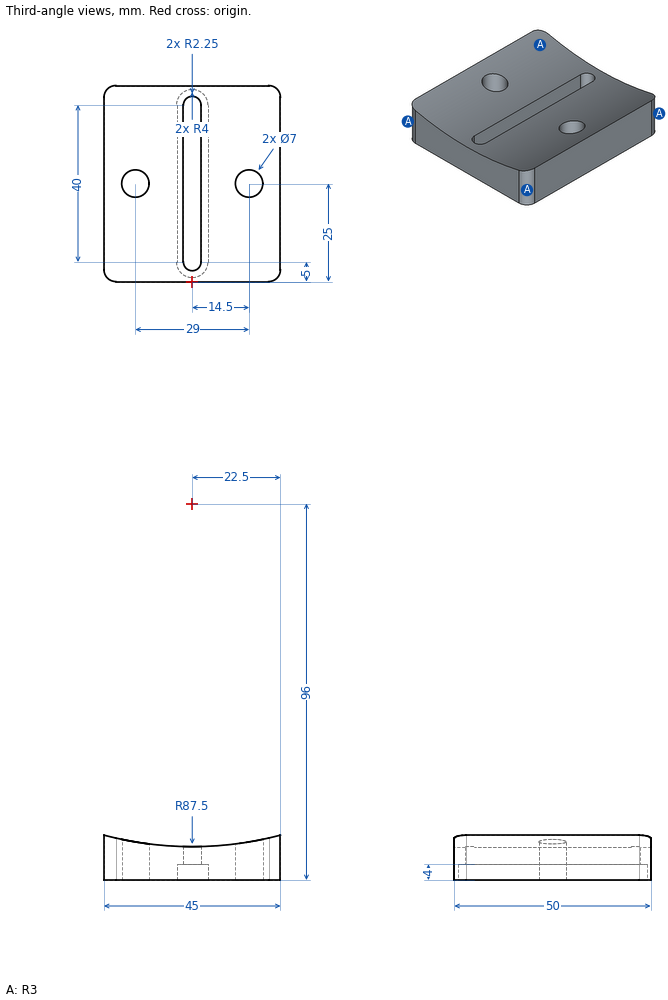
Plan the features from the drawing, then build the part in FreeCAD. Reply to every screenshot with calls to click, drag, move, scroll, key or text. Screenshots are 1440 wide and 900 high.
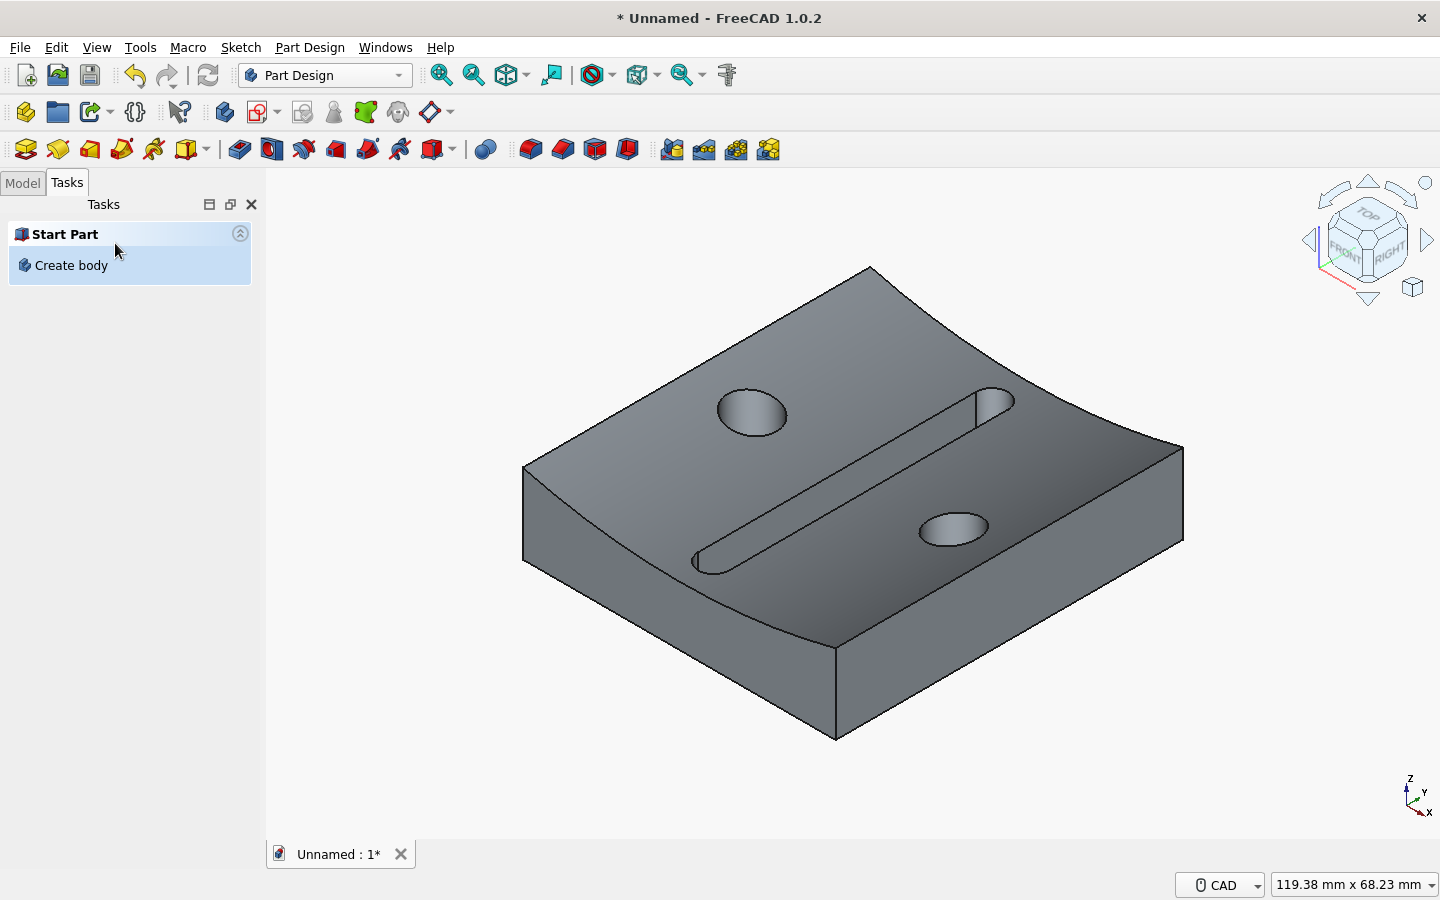
click(836, 693)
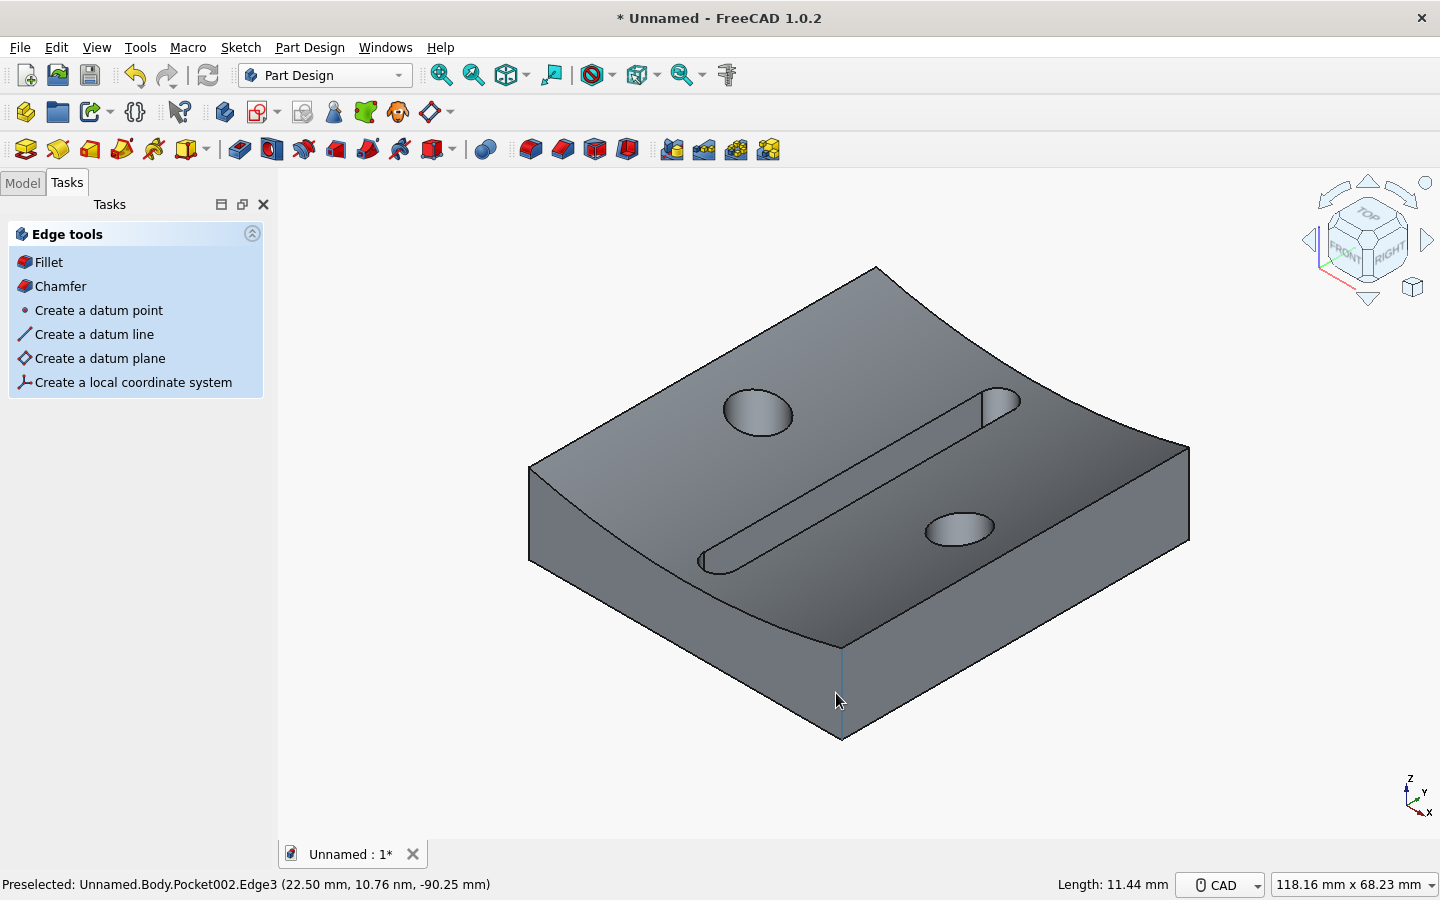
key(2)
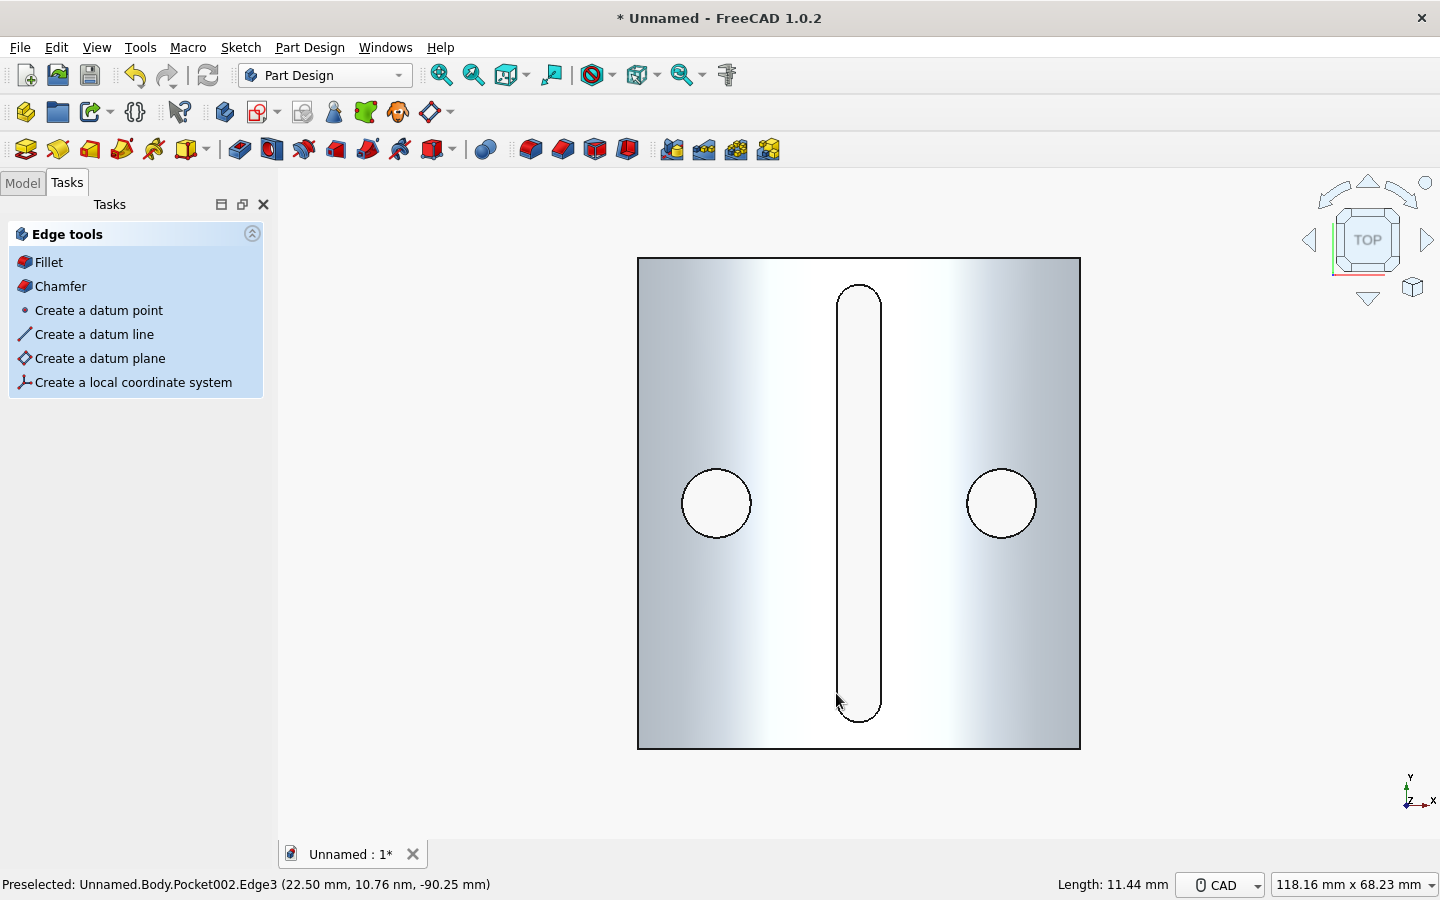
key(1)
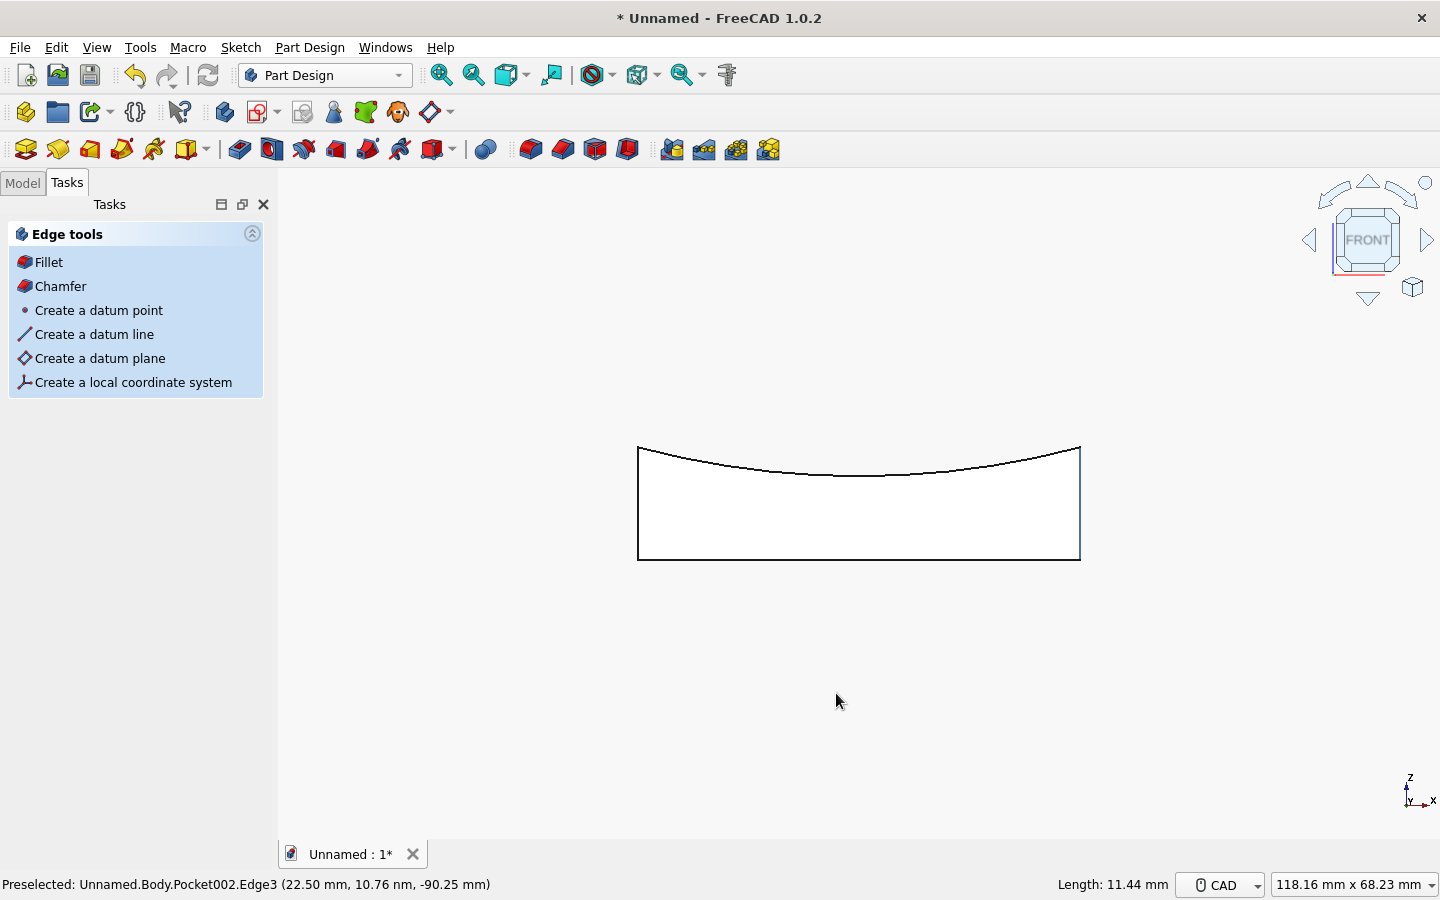
click(442, 76)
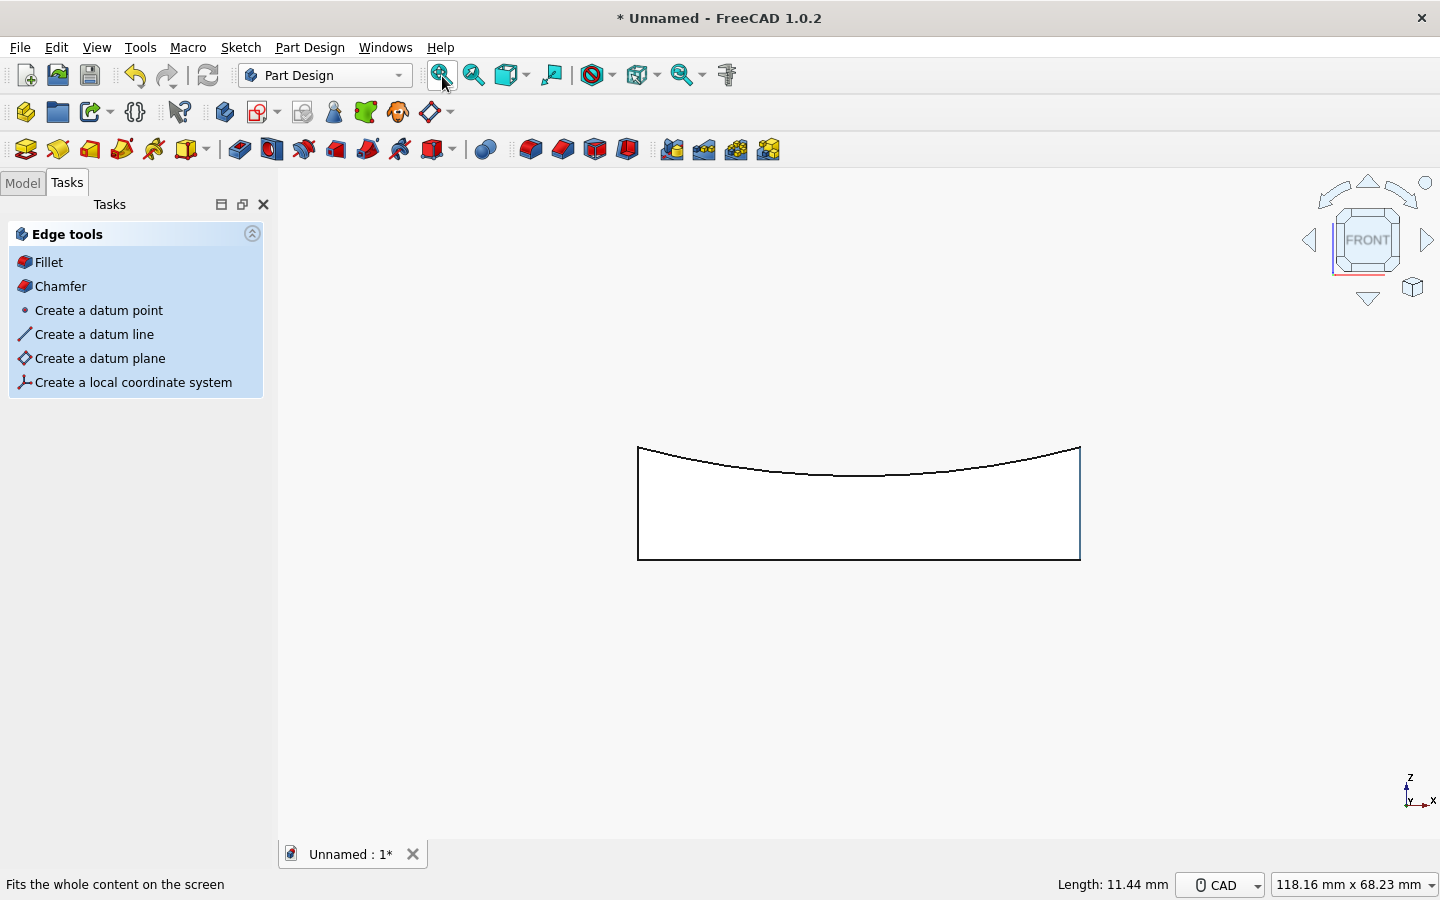
click(638, 502, ctrl)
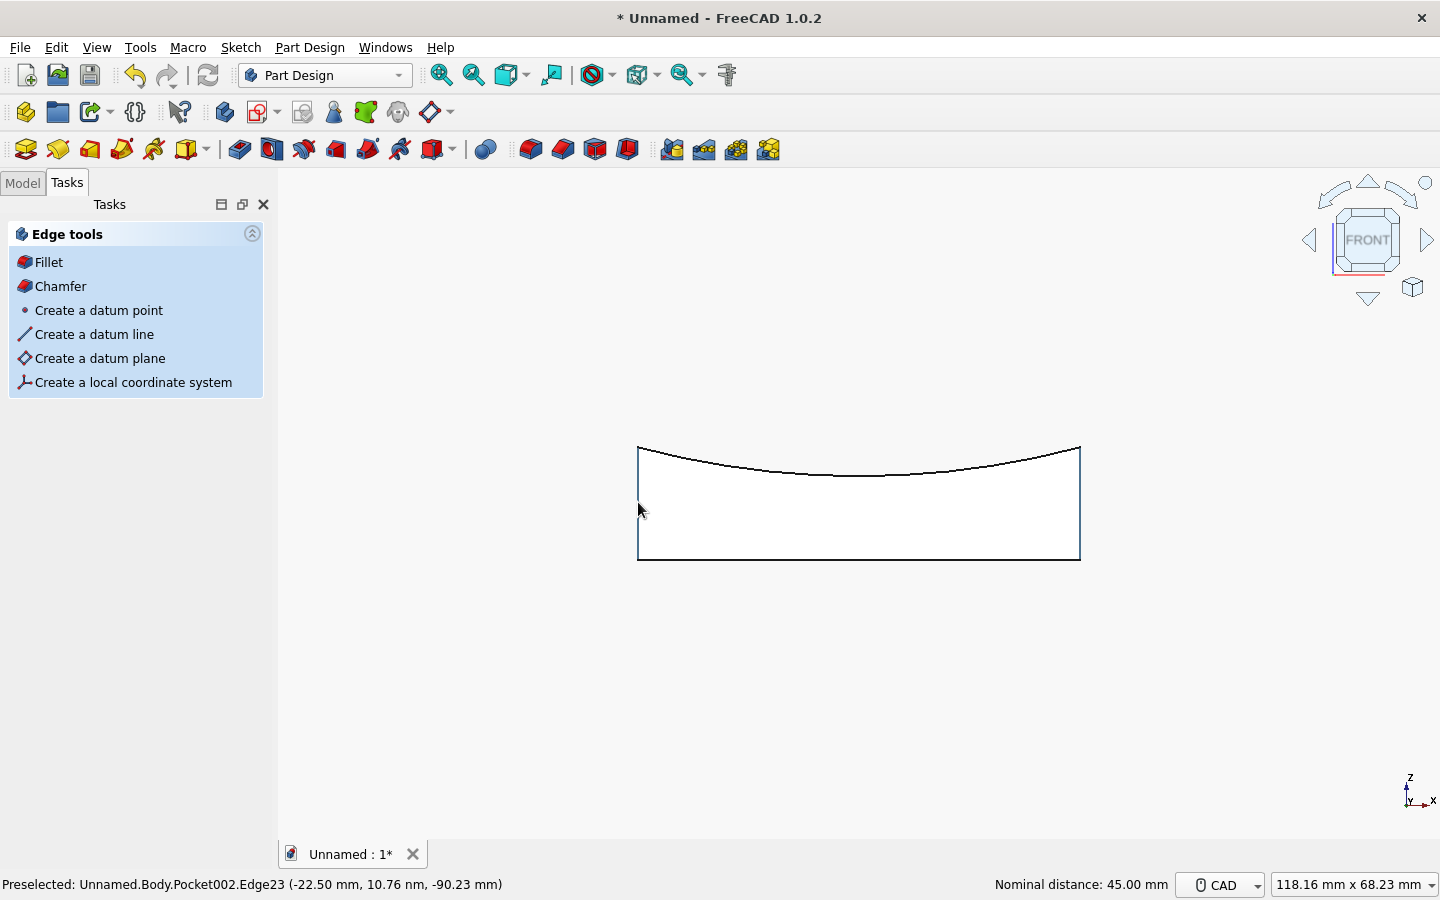
key(3)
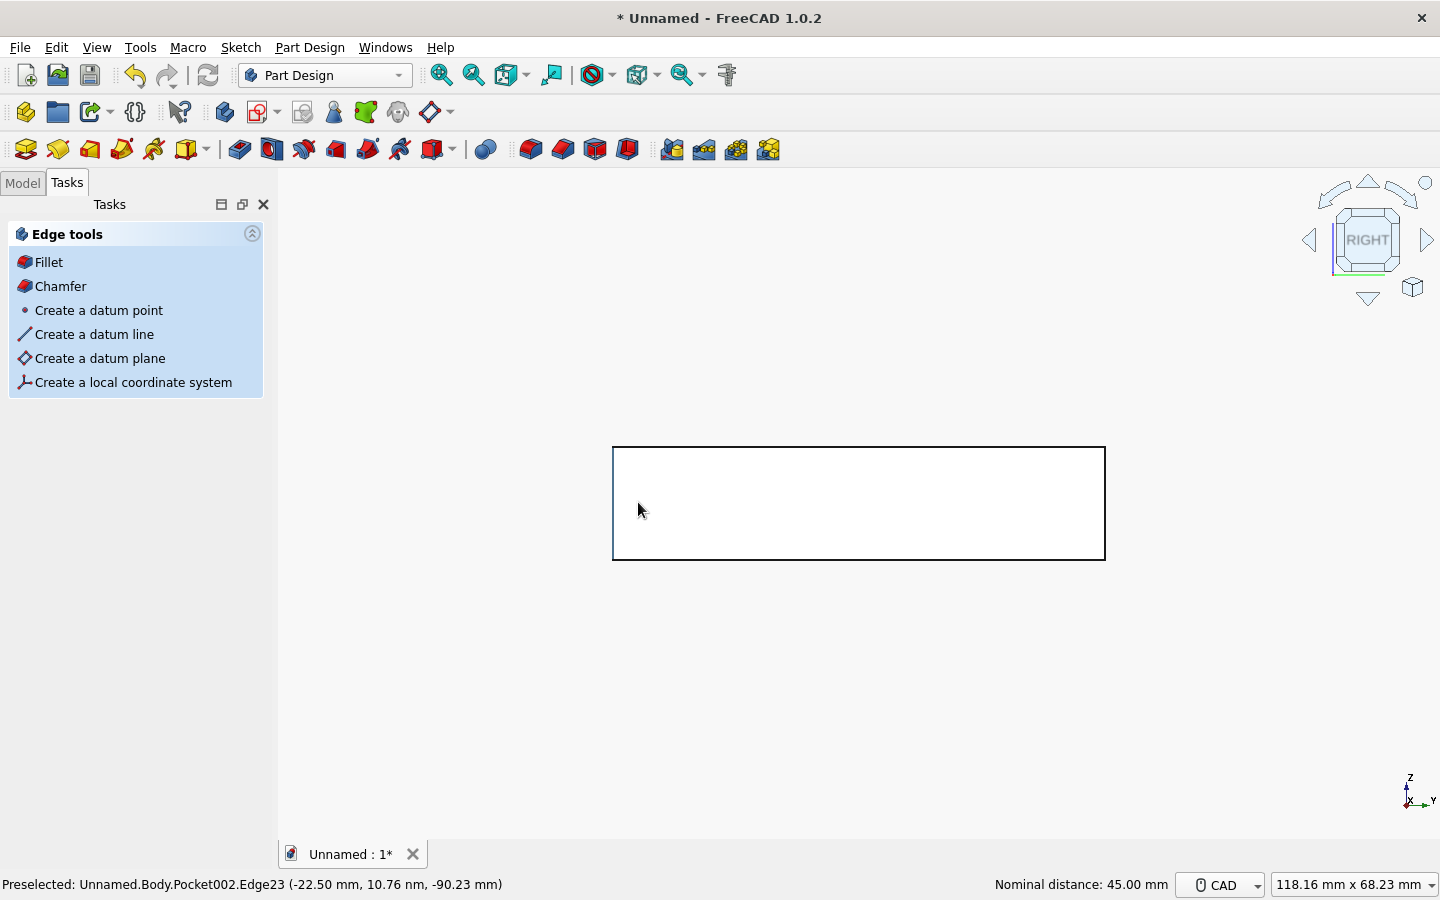
click(442, 76)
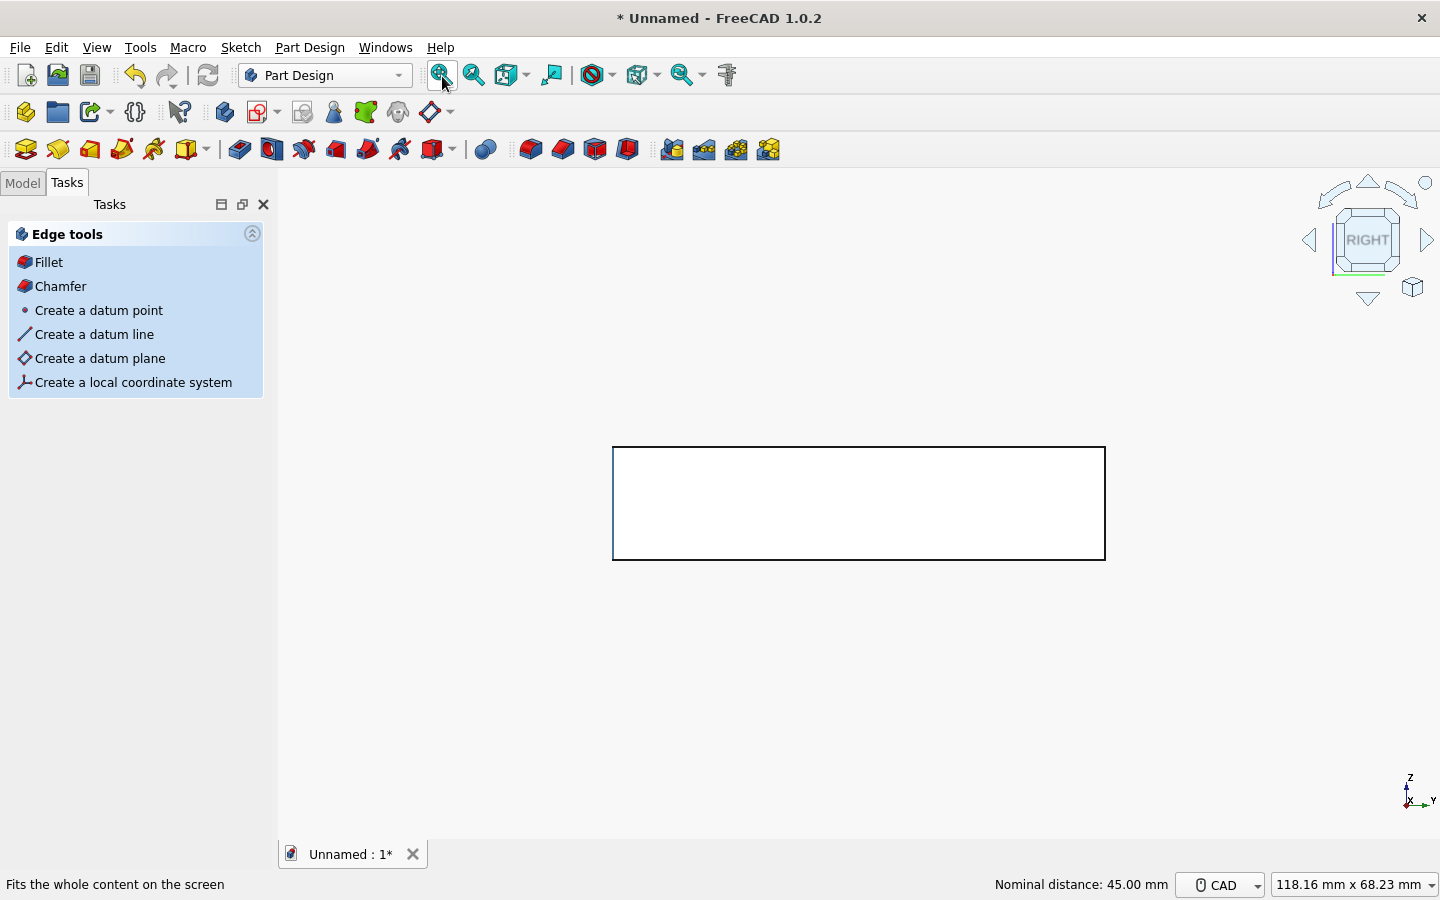
click(1105, 502, ctrl)